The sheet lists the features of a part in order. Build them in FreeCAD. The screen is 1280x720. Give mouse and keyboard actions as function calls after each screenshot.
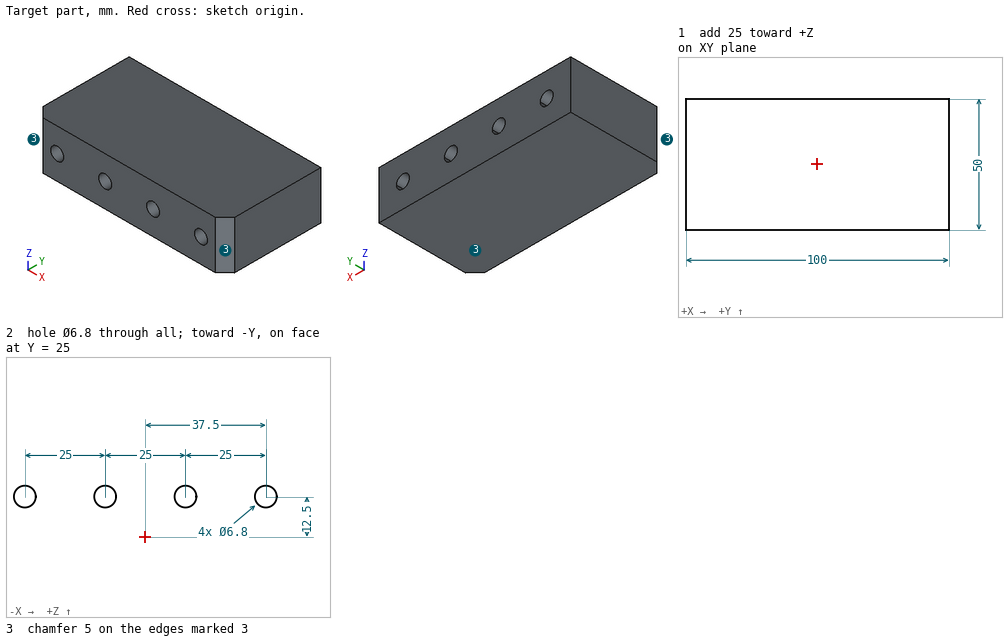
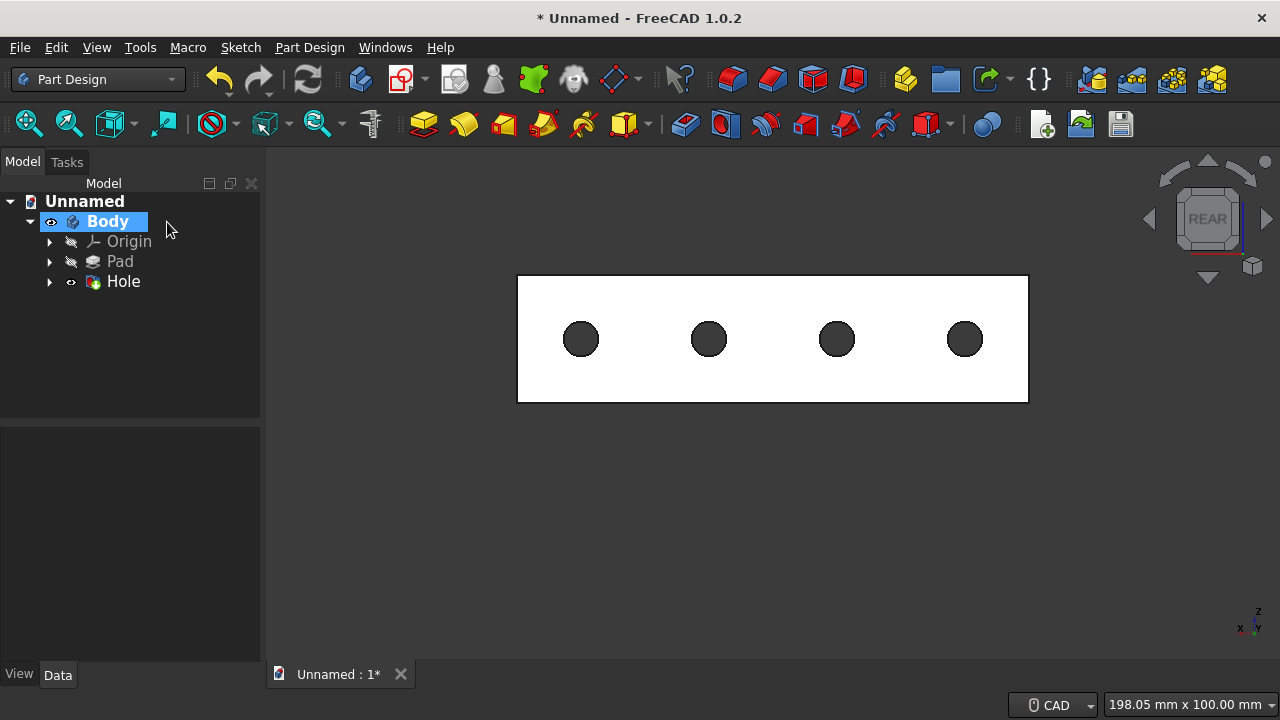
key(0)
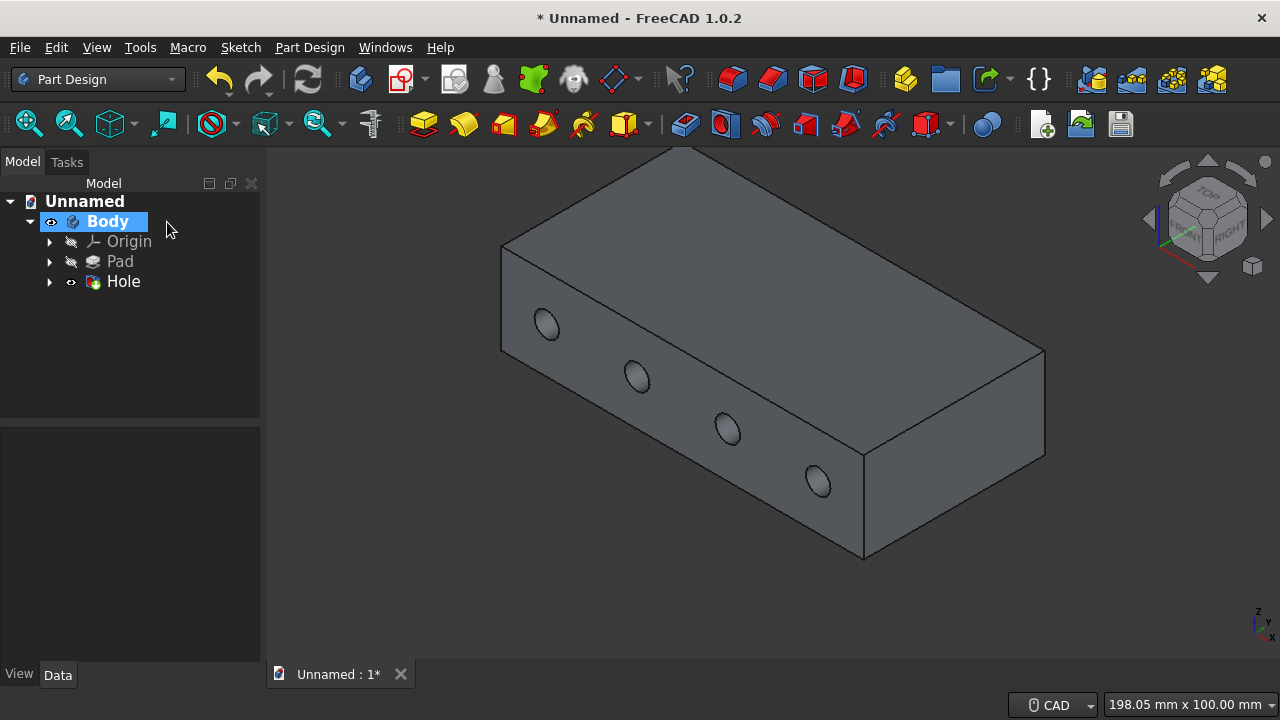
click(30, 124)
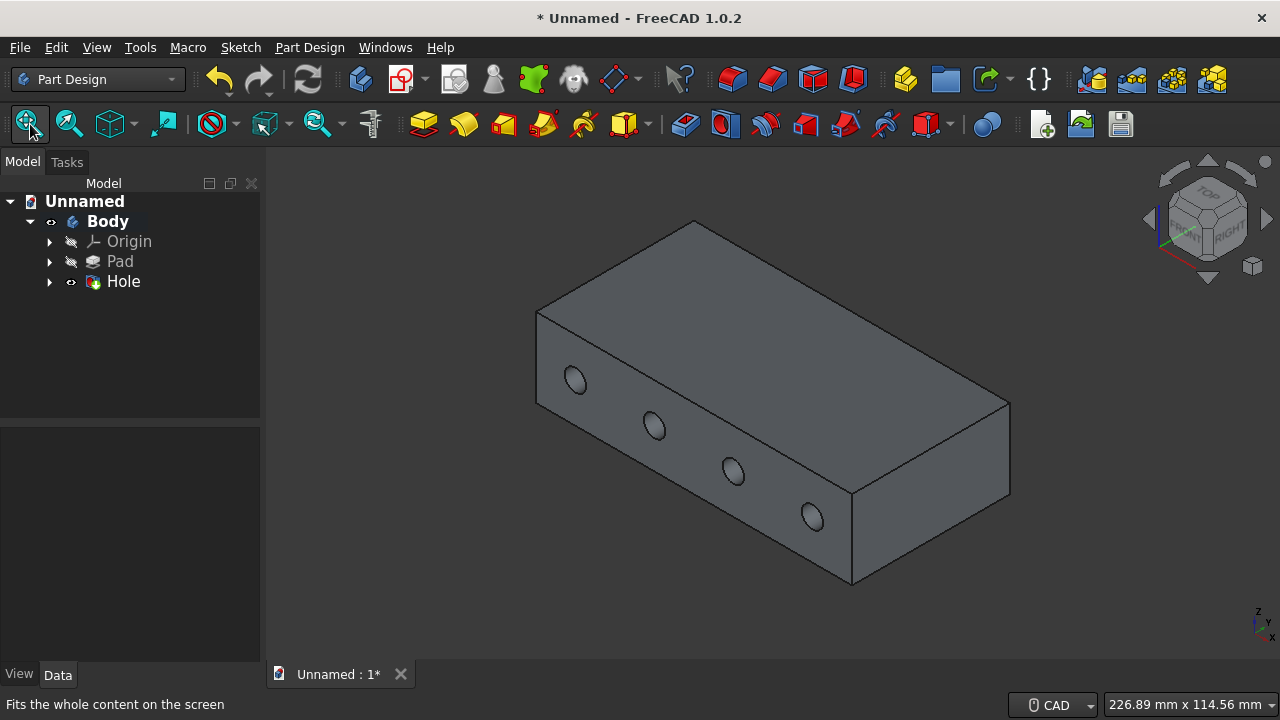
click(852, 539)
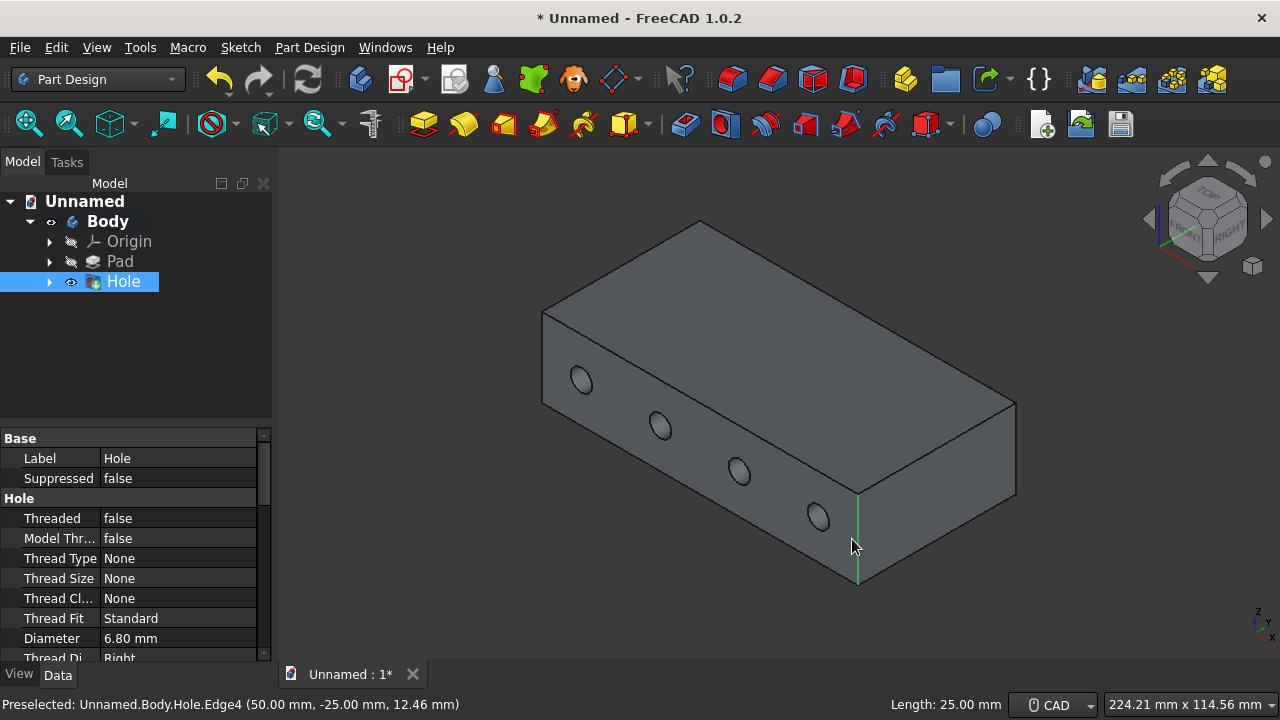
key(2)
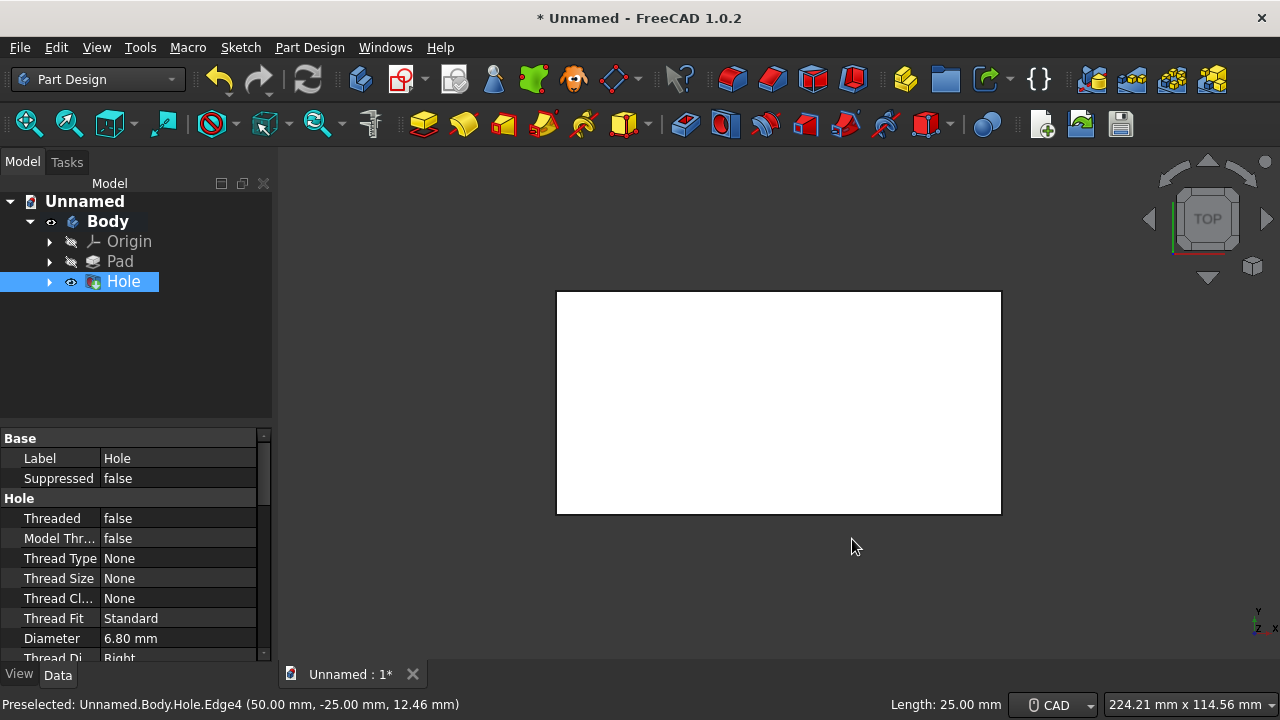
click(30, 124)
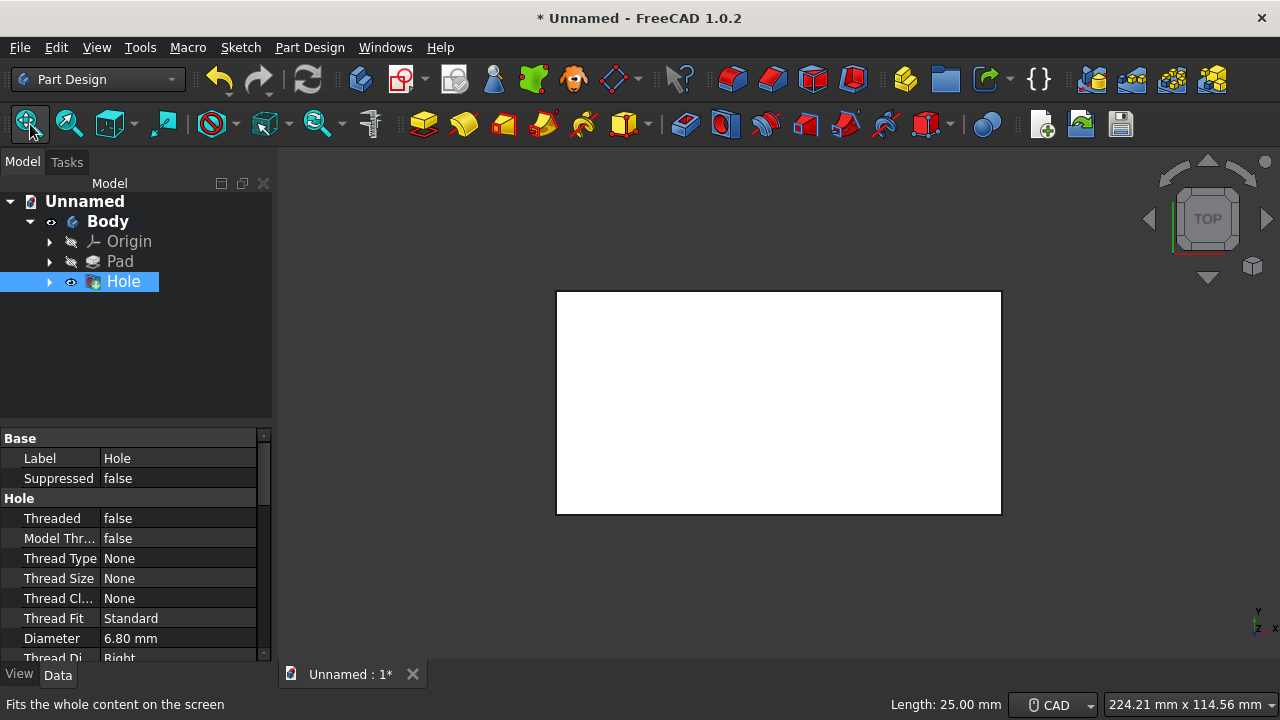
key(1)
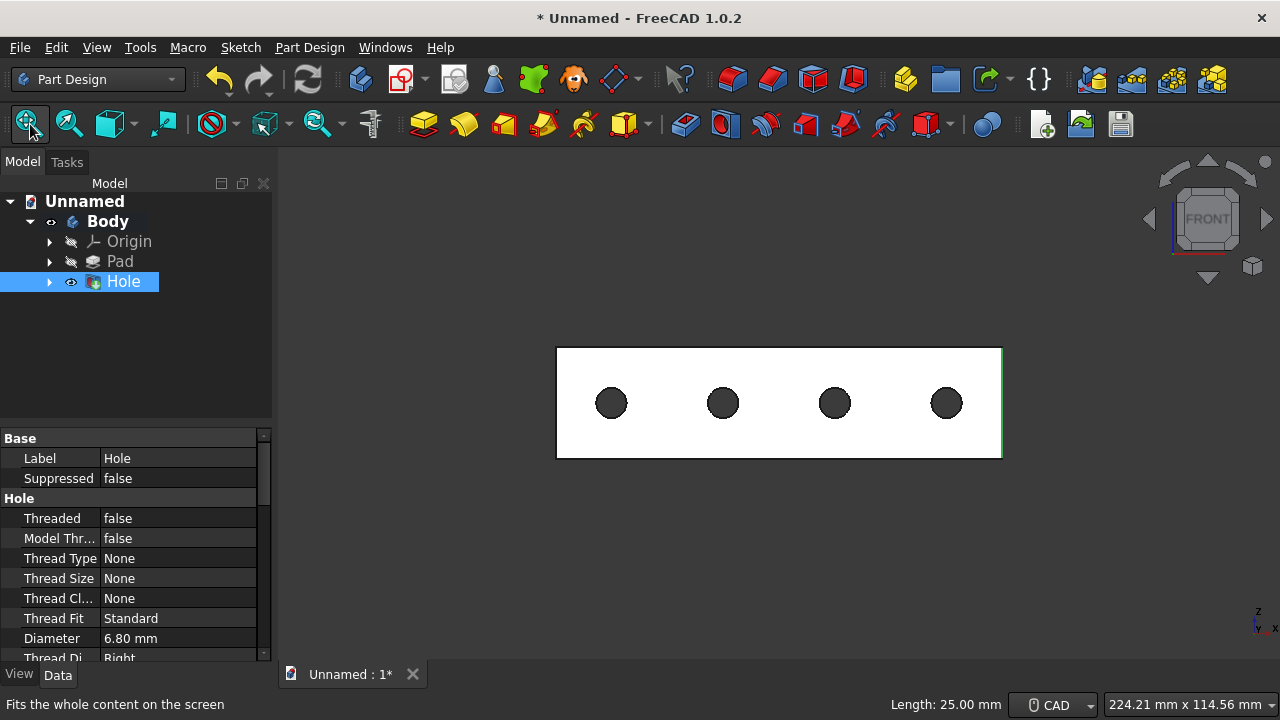
click(30, 124)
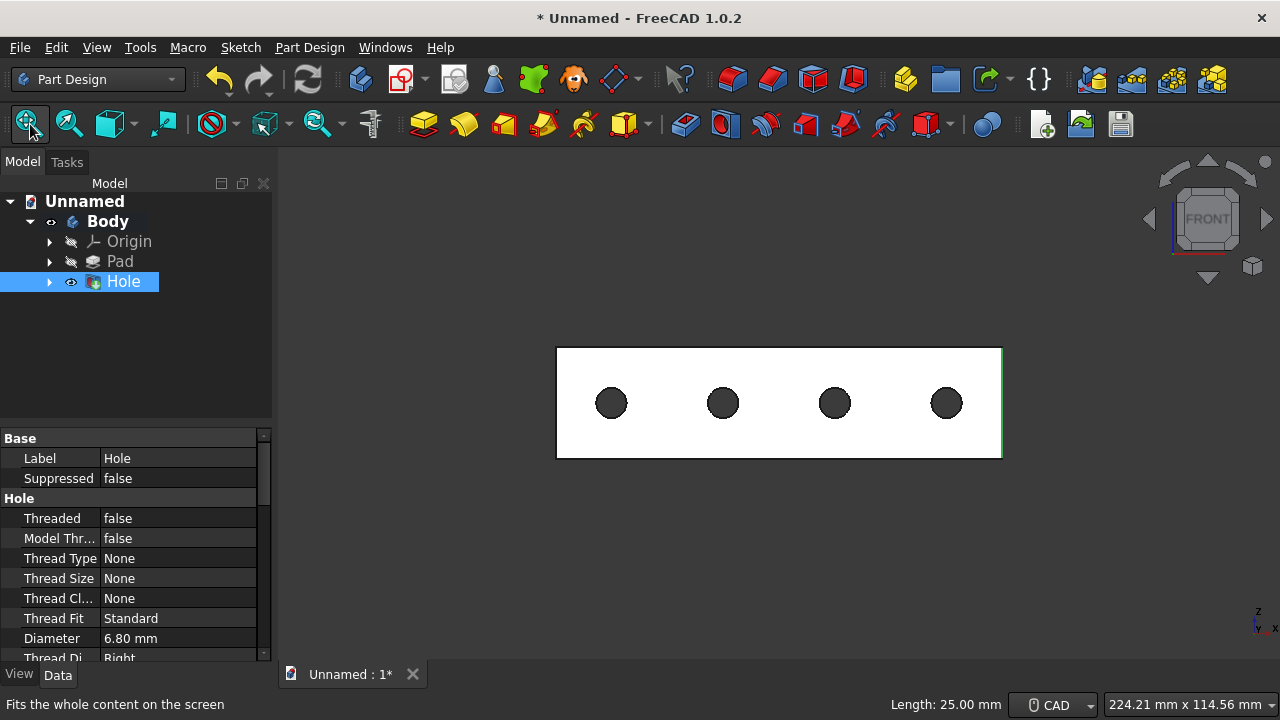
click(556, 402, ctrl)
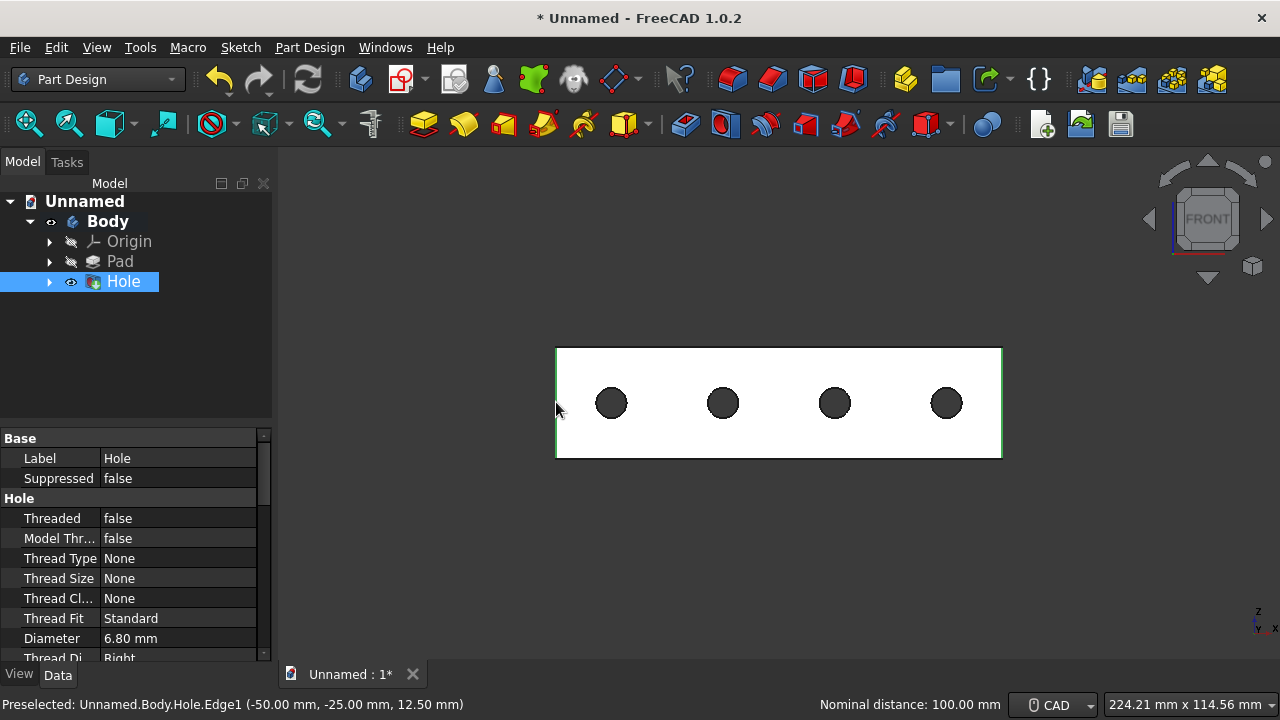
click(774, 80)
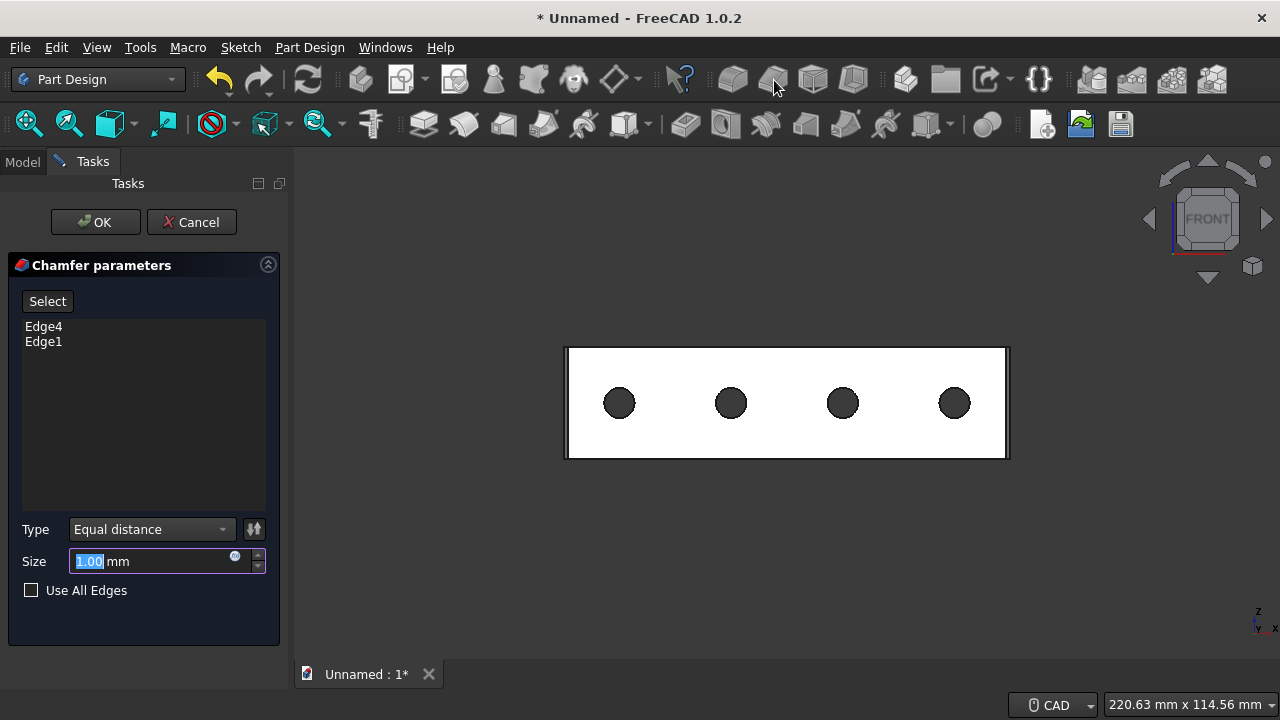
text(5)
key(Tab)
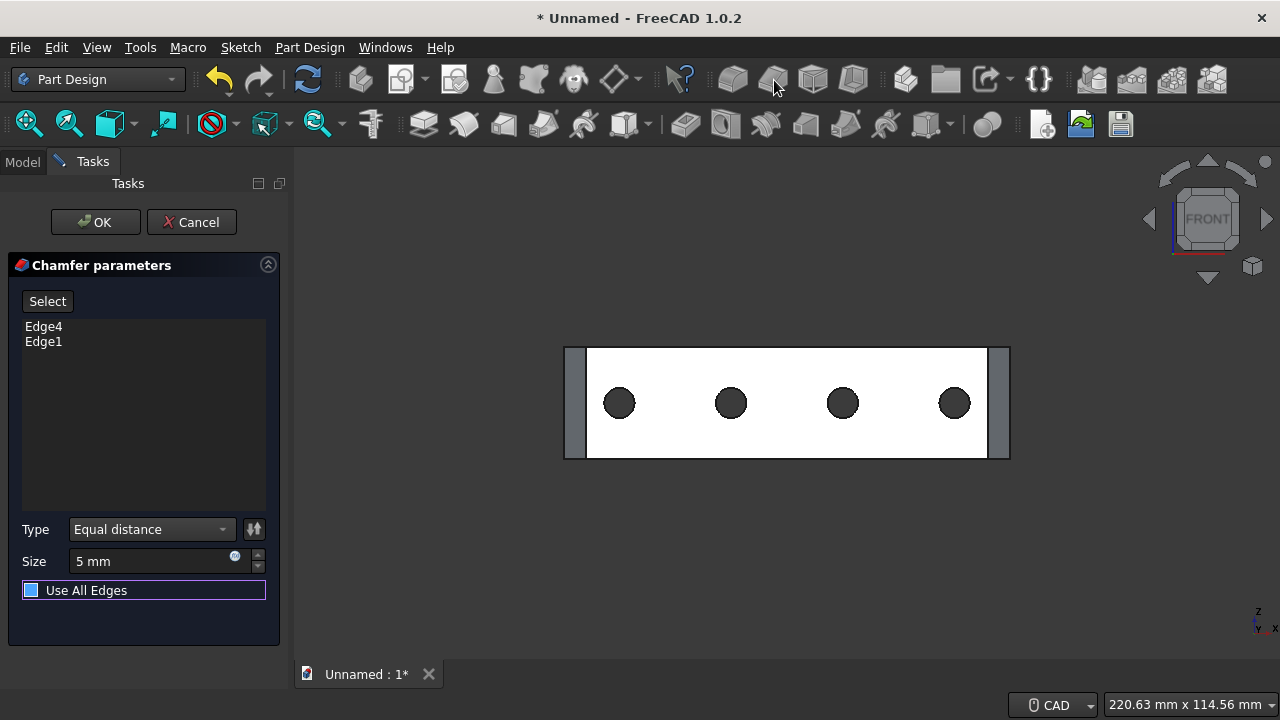
click(96, 222)